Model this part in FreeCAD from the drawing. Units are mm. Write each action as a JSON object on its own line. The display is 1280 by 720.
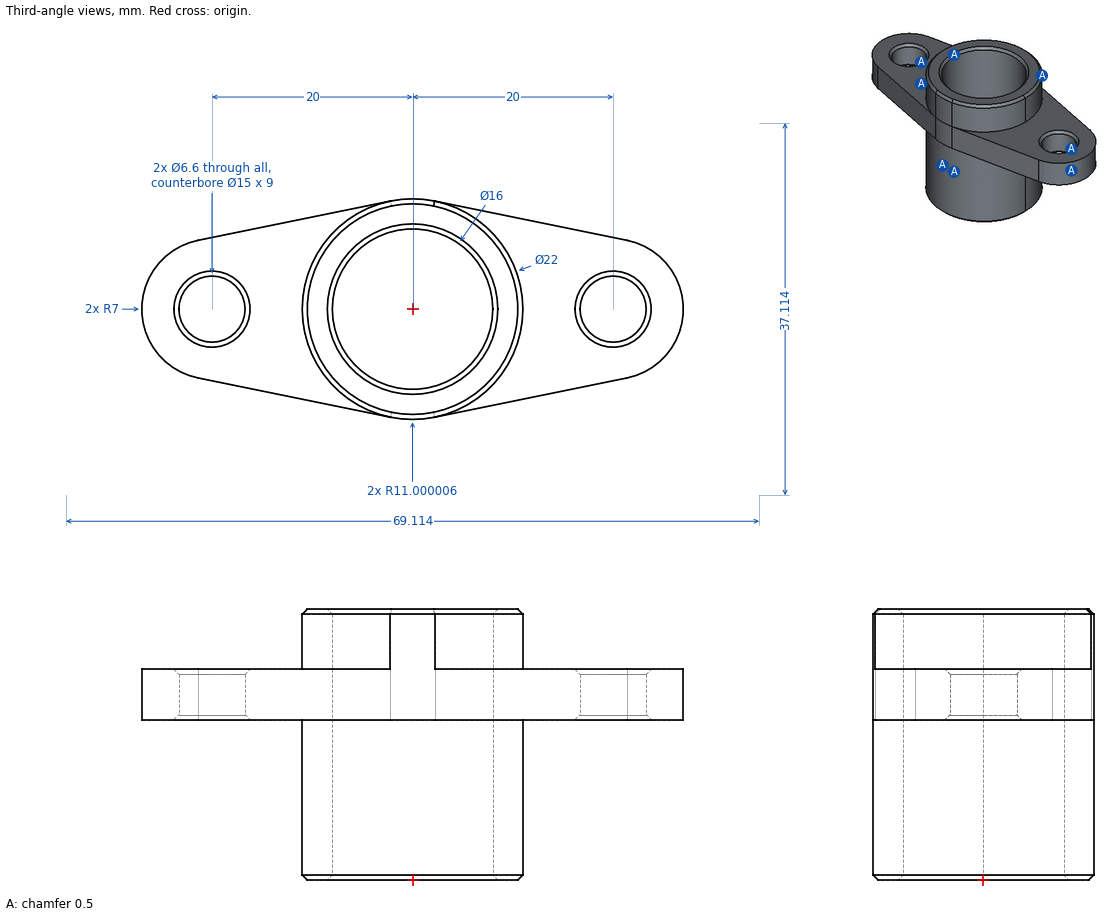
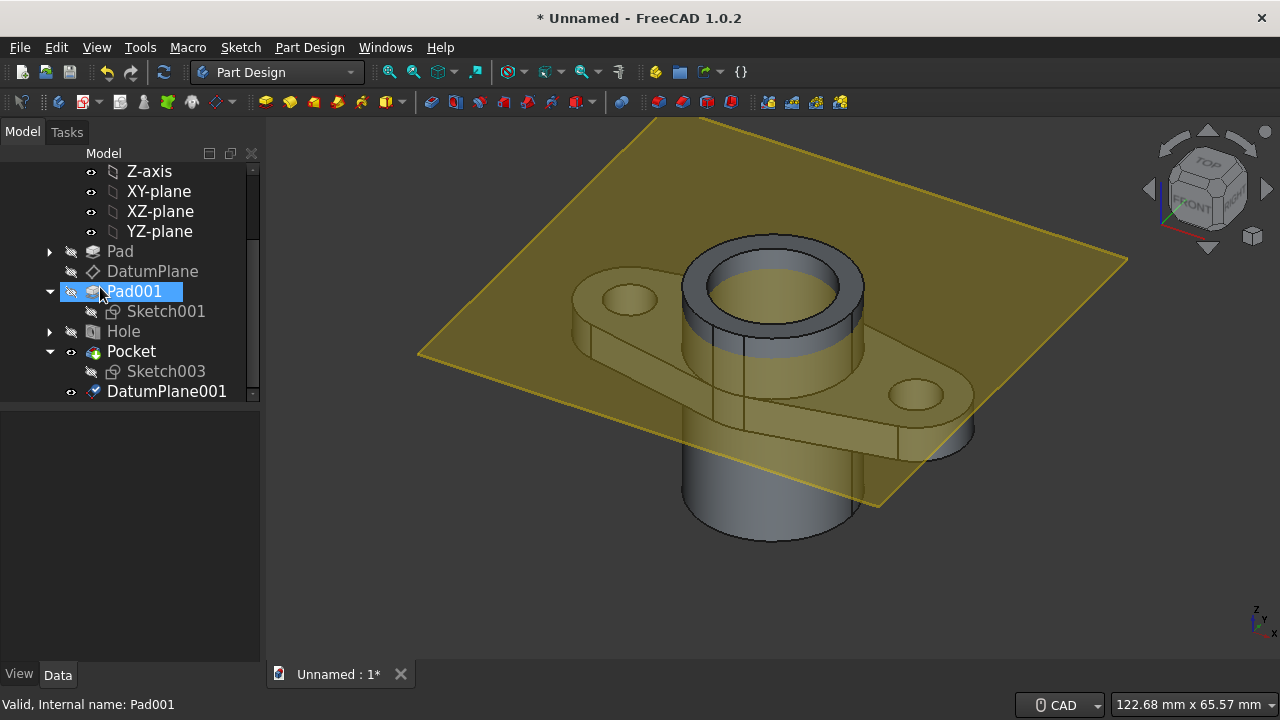
{"action": "left_click", "coordinate": [116, 392]}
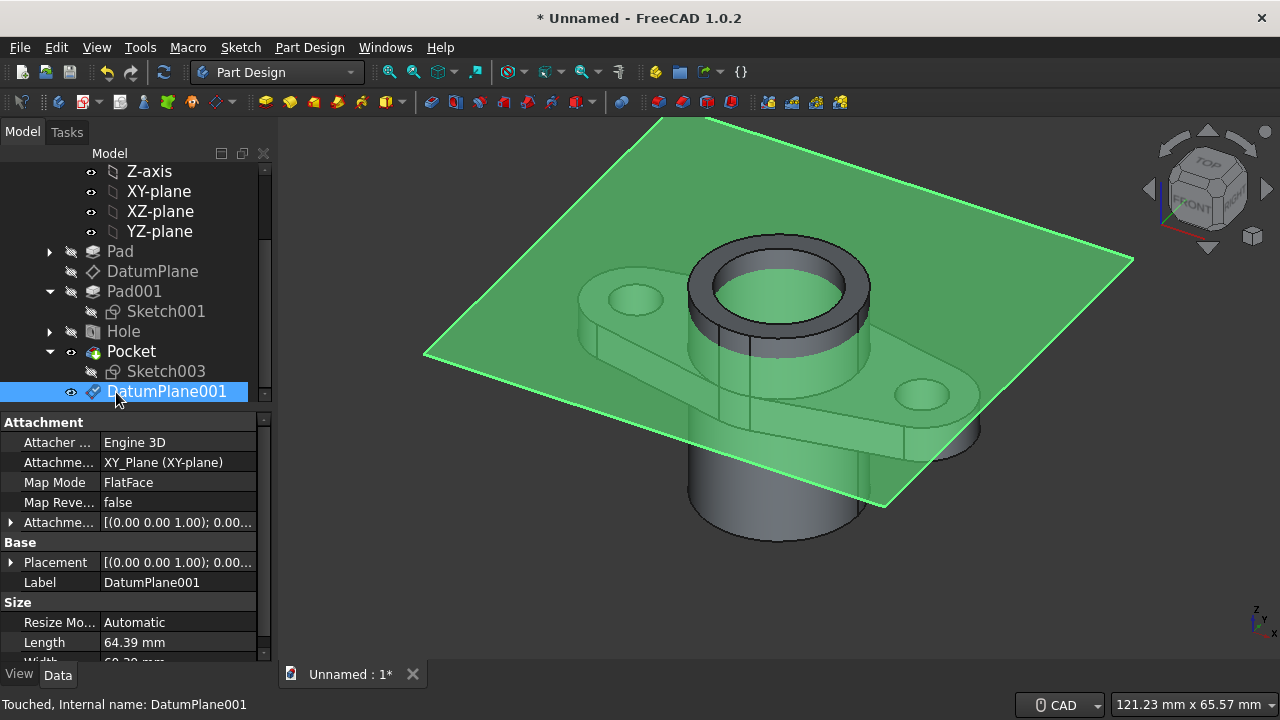
{"action": "left_click", "coordinate": [84, 102]}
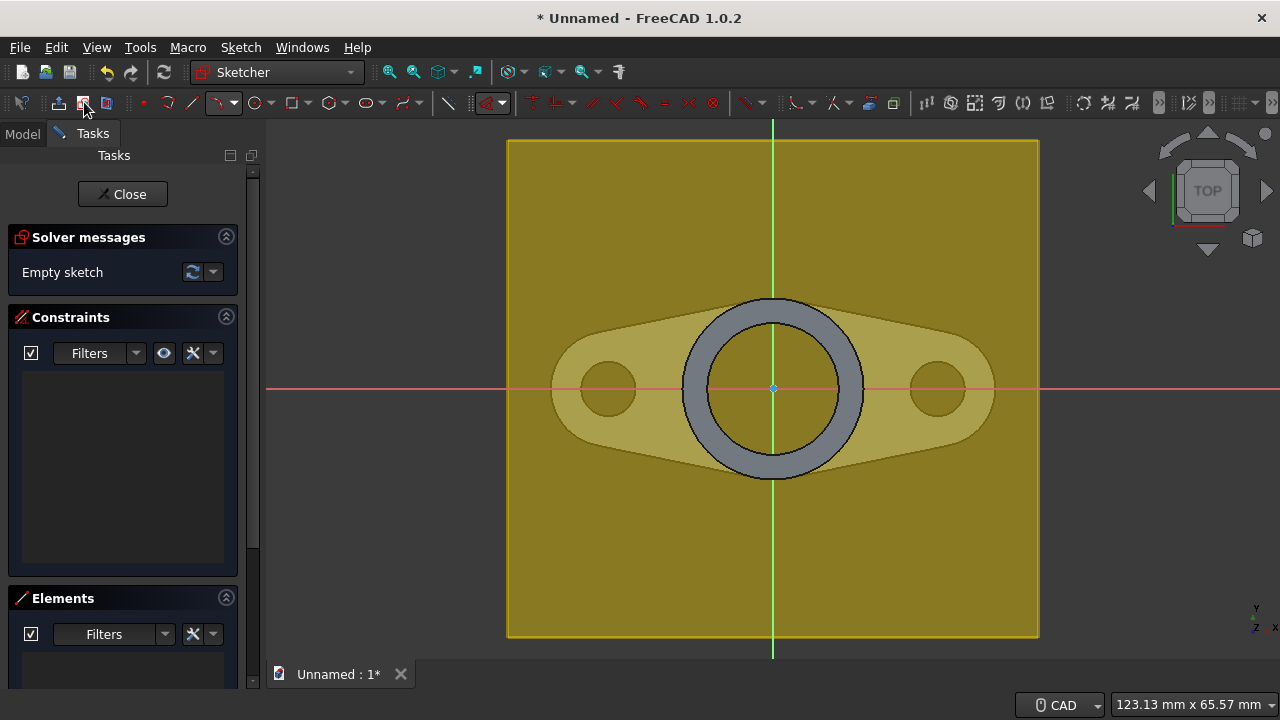
{"action": "key", "text": "q s"}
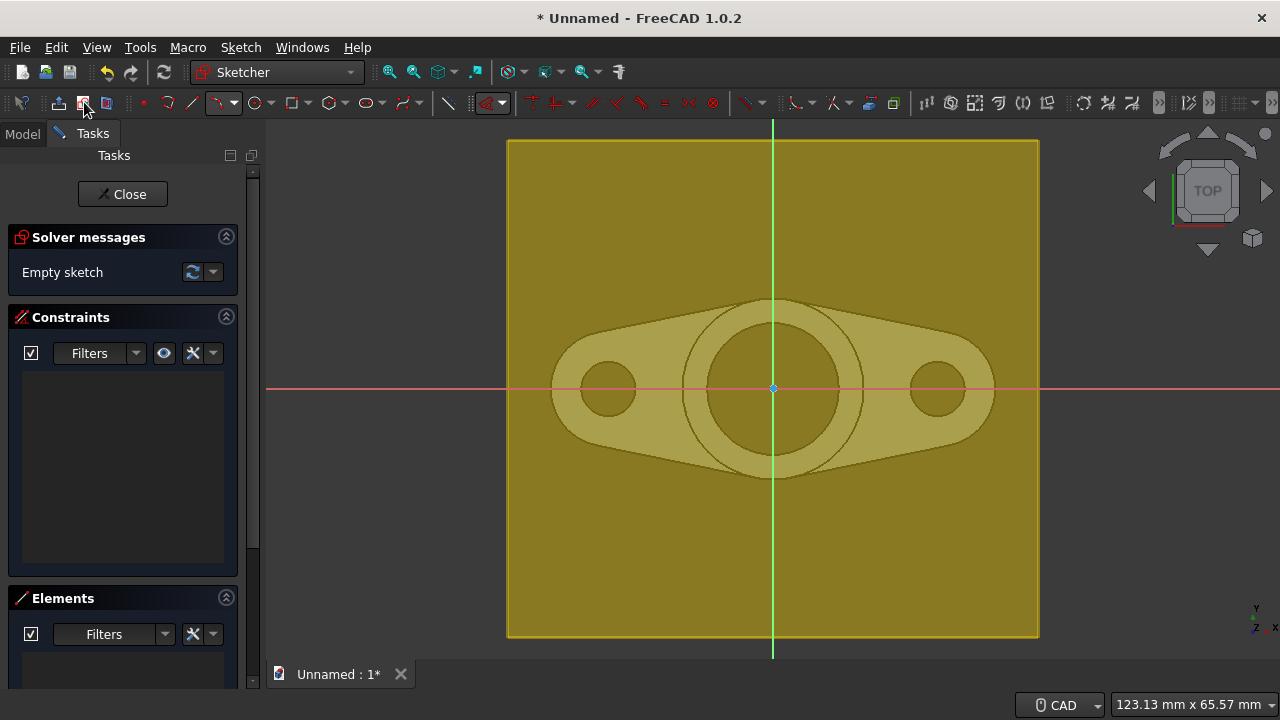
{"action": "scroll", "coordinate": [856, 389], "scroll_direction": "up", "scroll_amount": 3}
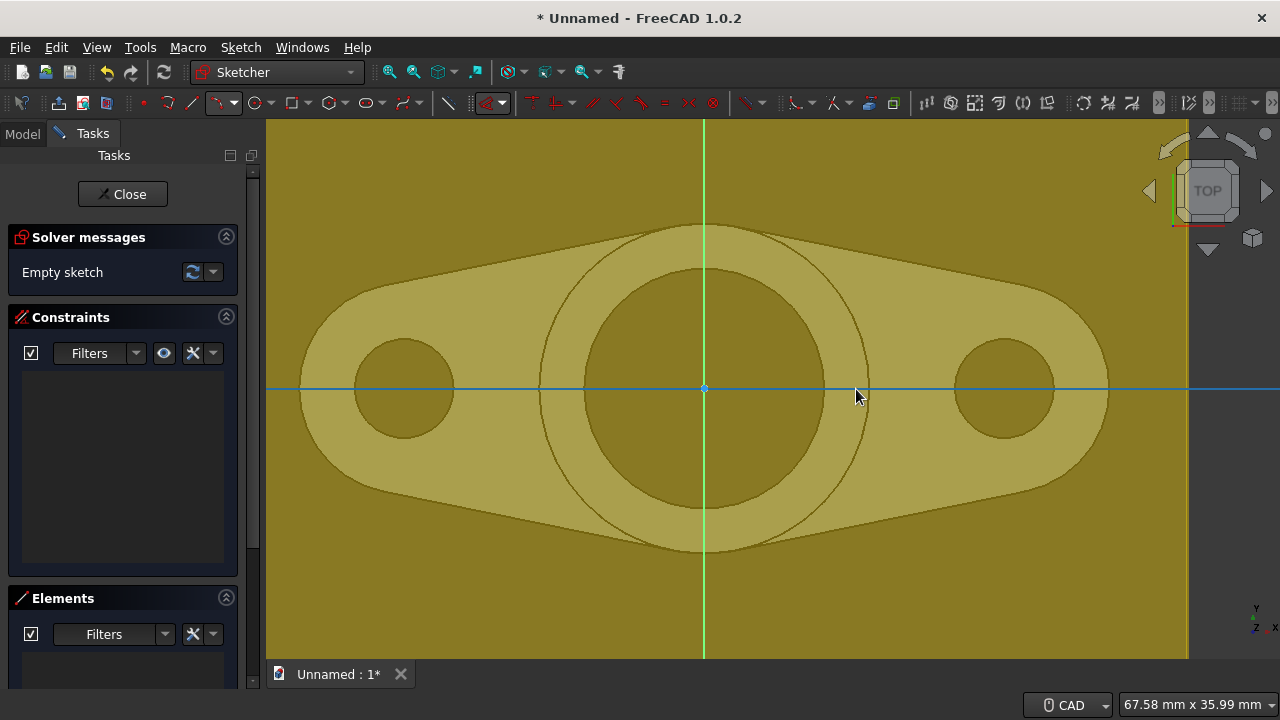
{"action": "left_click", "coordinate": [256, 104]}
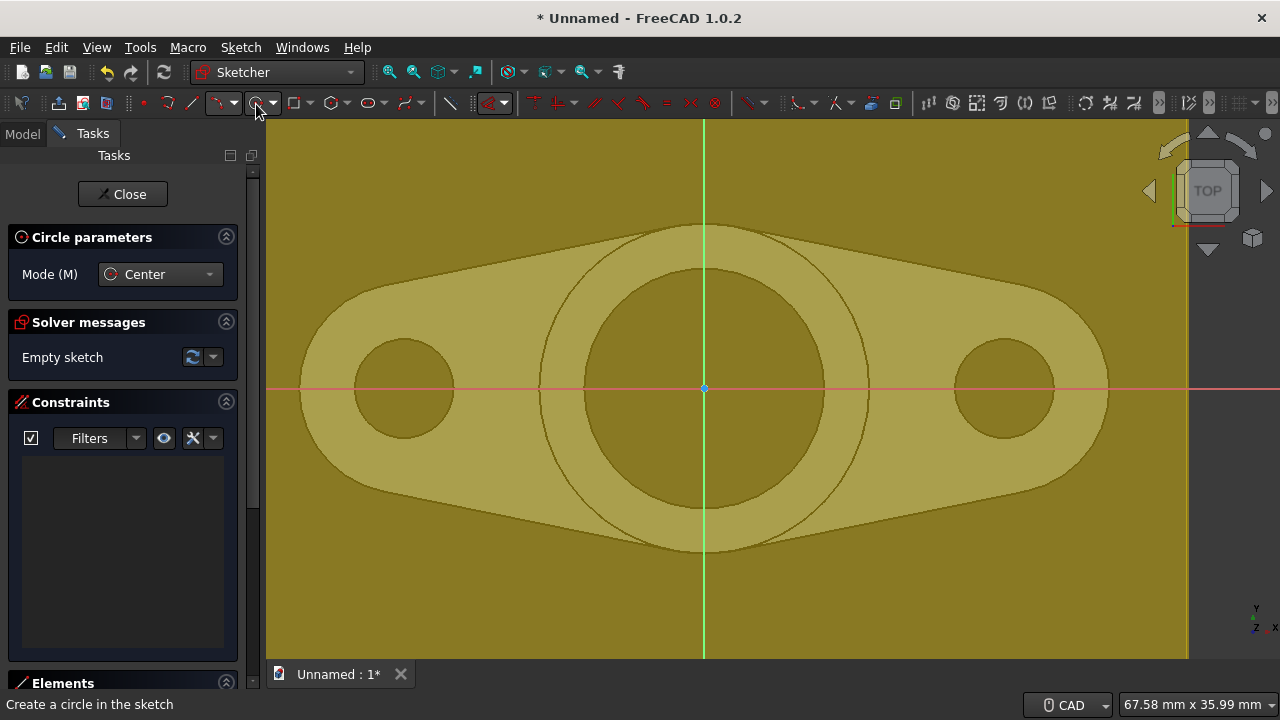
{"action": "left_click", "coordinate": [704, 389]}
{"action": "left_click", "coordinate": [821, 272]}
{"action": "key", "text": "Escape"}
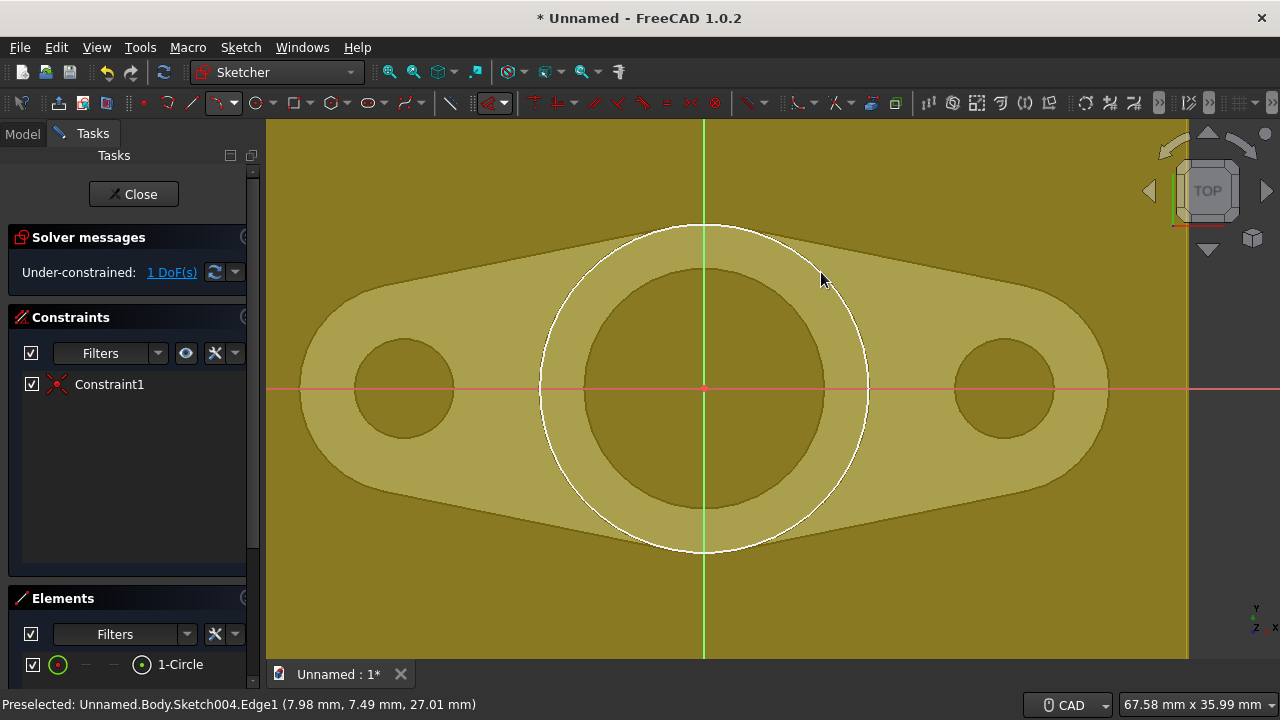
{"action": "left_click", "coordinate": [820, 272]}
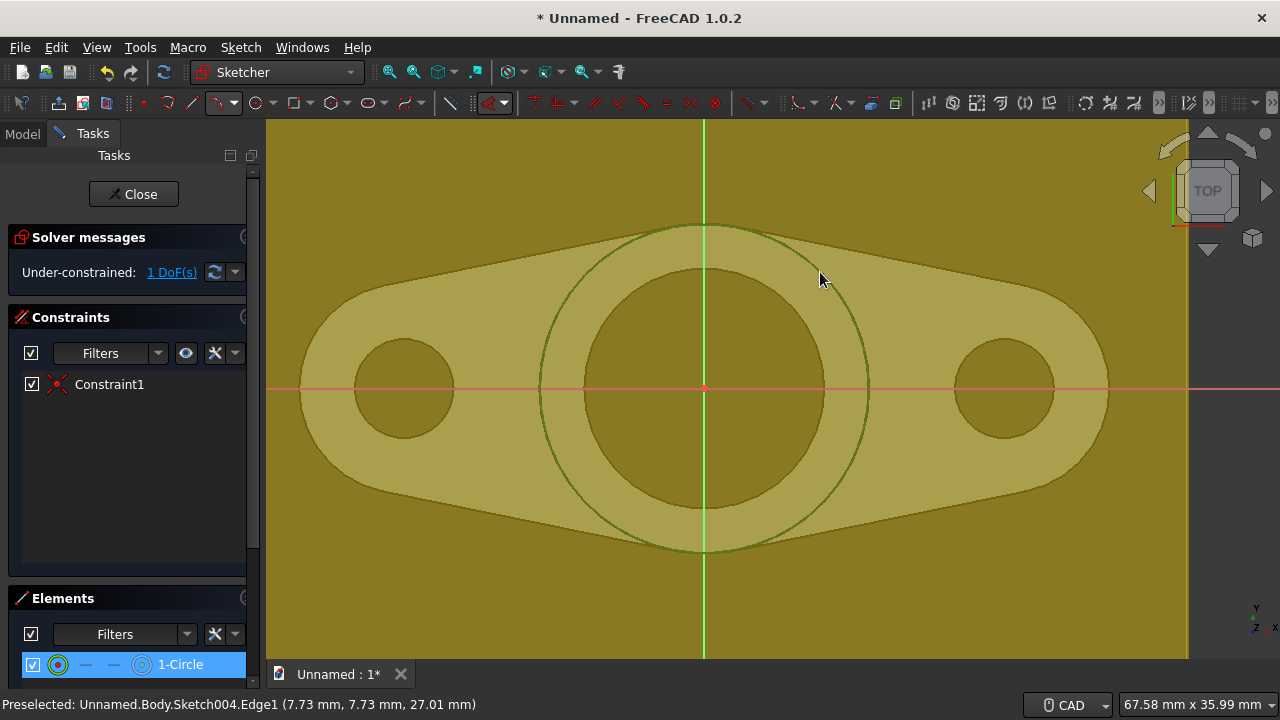
{"action": "left_click", "coordinate": [506, 104]}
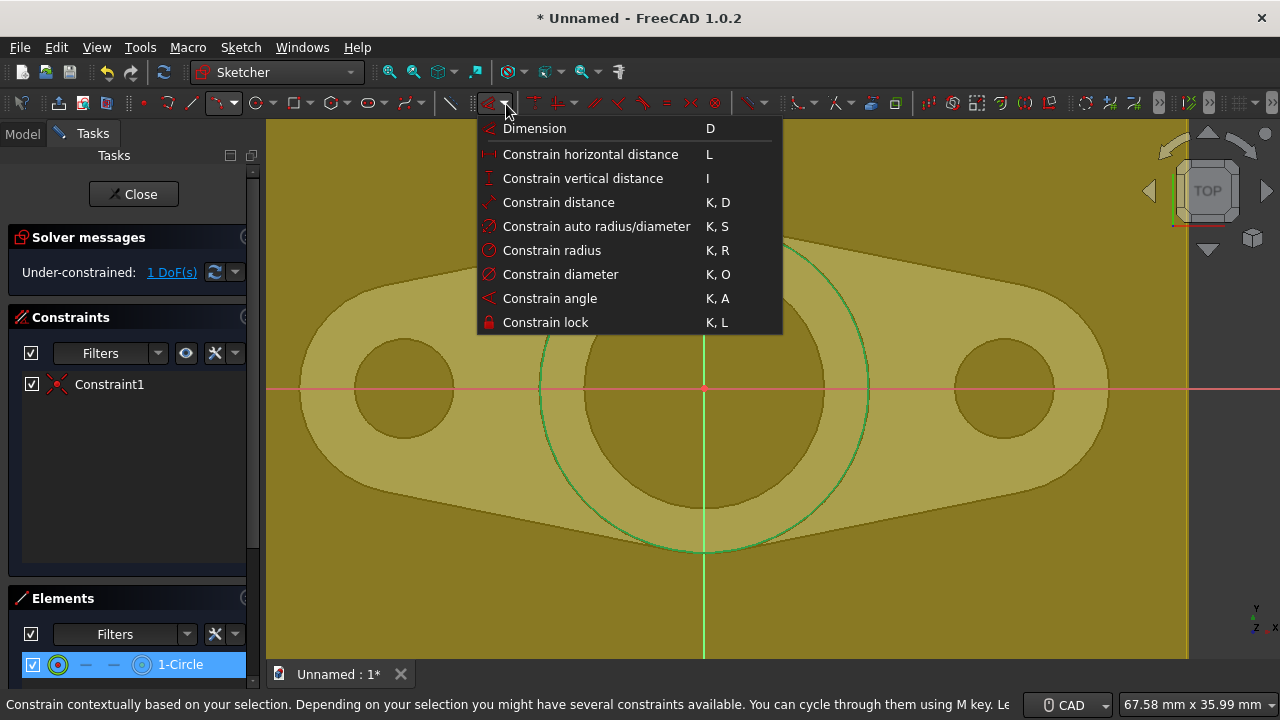
{"action": "left_click", "coordinate": [630, 274]}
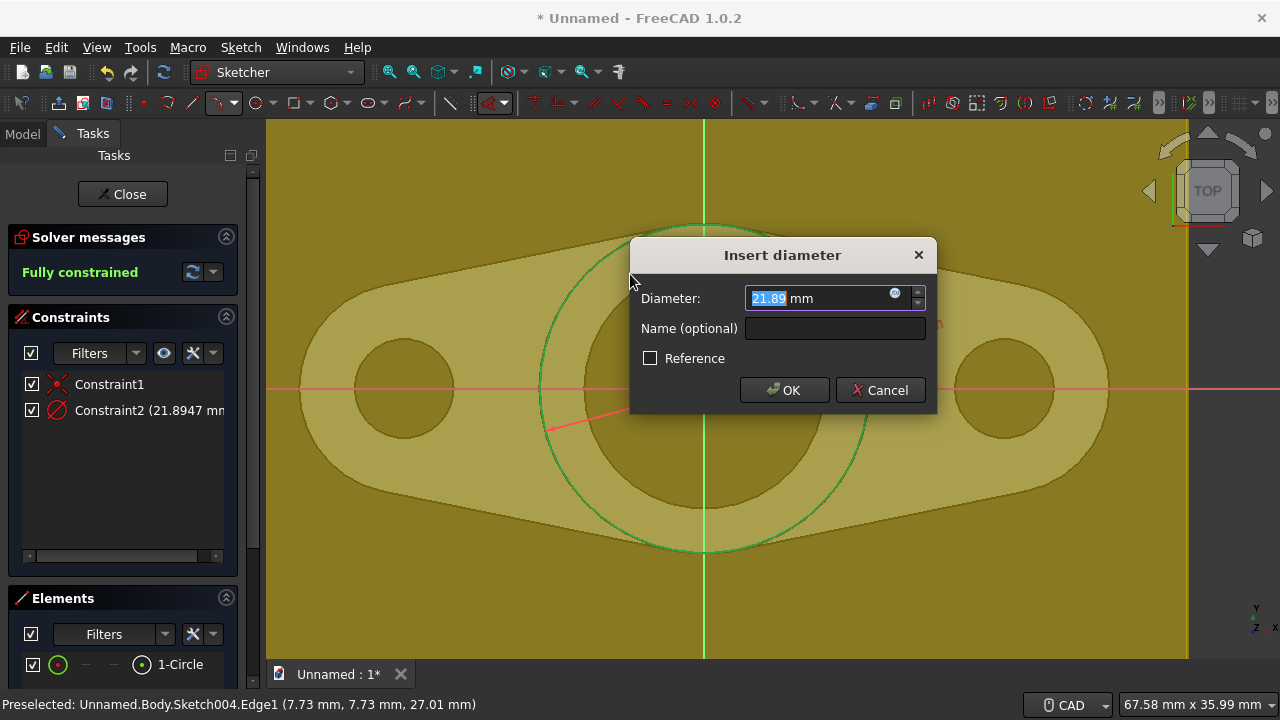
{"action": "type", "text": "22"}
{"action": "key", "text": "Return"}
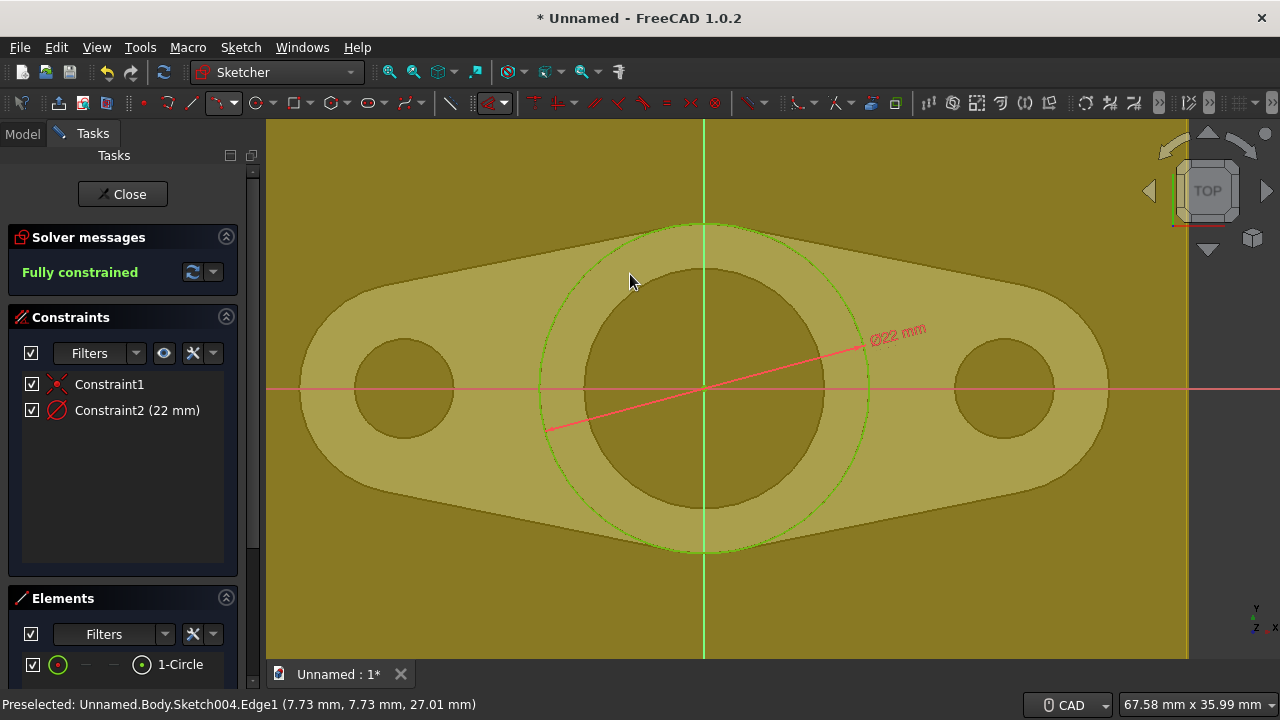
{"action": "left_click", "coordinate": [123, 194]}